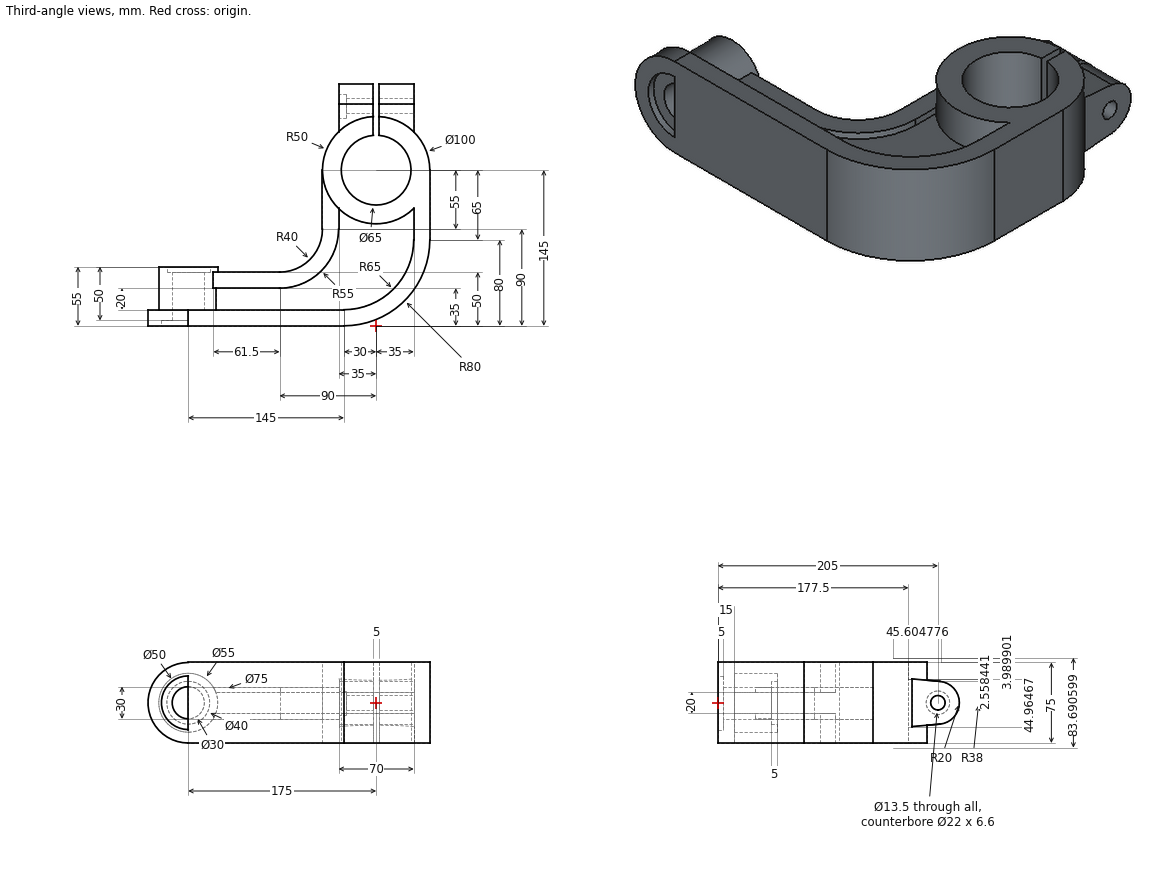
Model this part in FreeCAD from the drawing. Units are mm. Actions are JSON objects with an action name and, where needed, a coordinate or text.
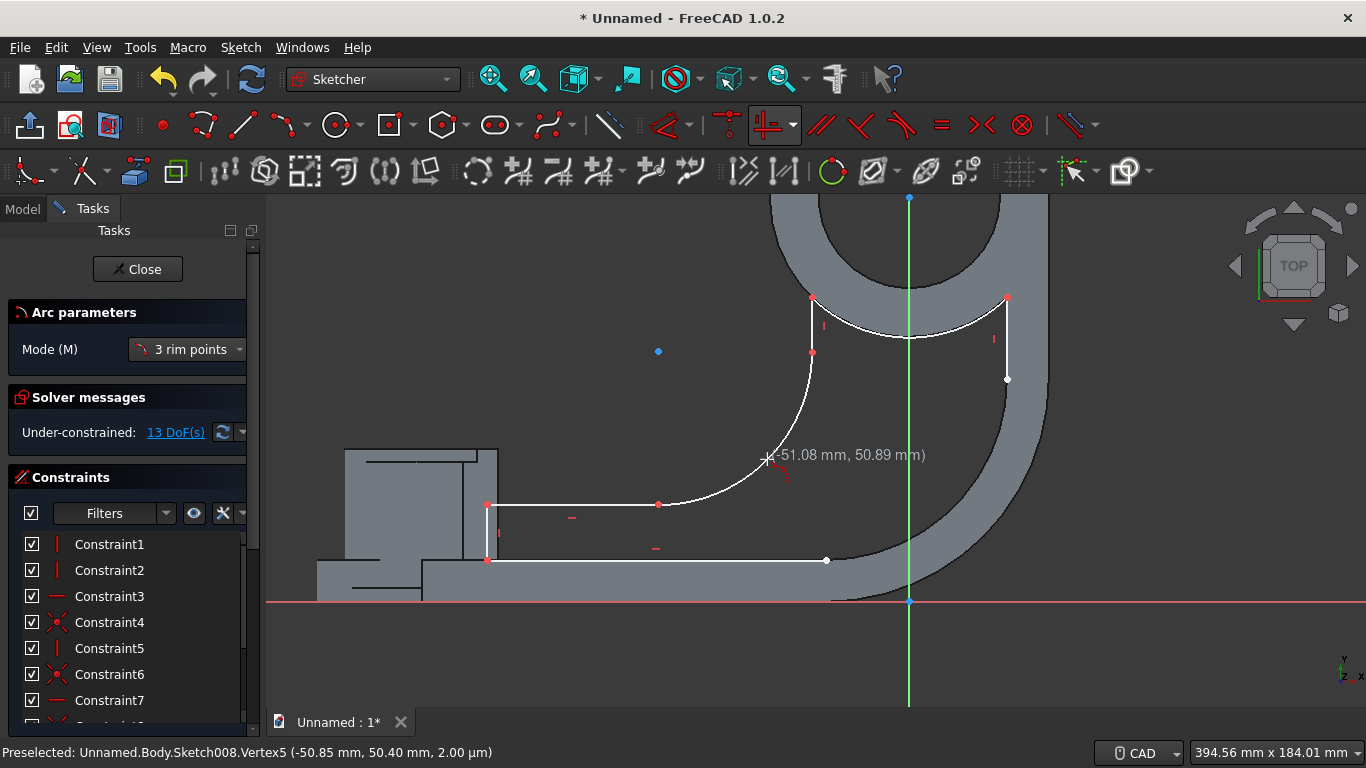
{"action": "left_click", "coordinate": [826, 561]}
{"action": "left_click", "coordinate": [1007, 380]}
{"action": "left_click", "coordinate": [954, 507]}
{"action": "key", "text": "Escape"}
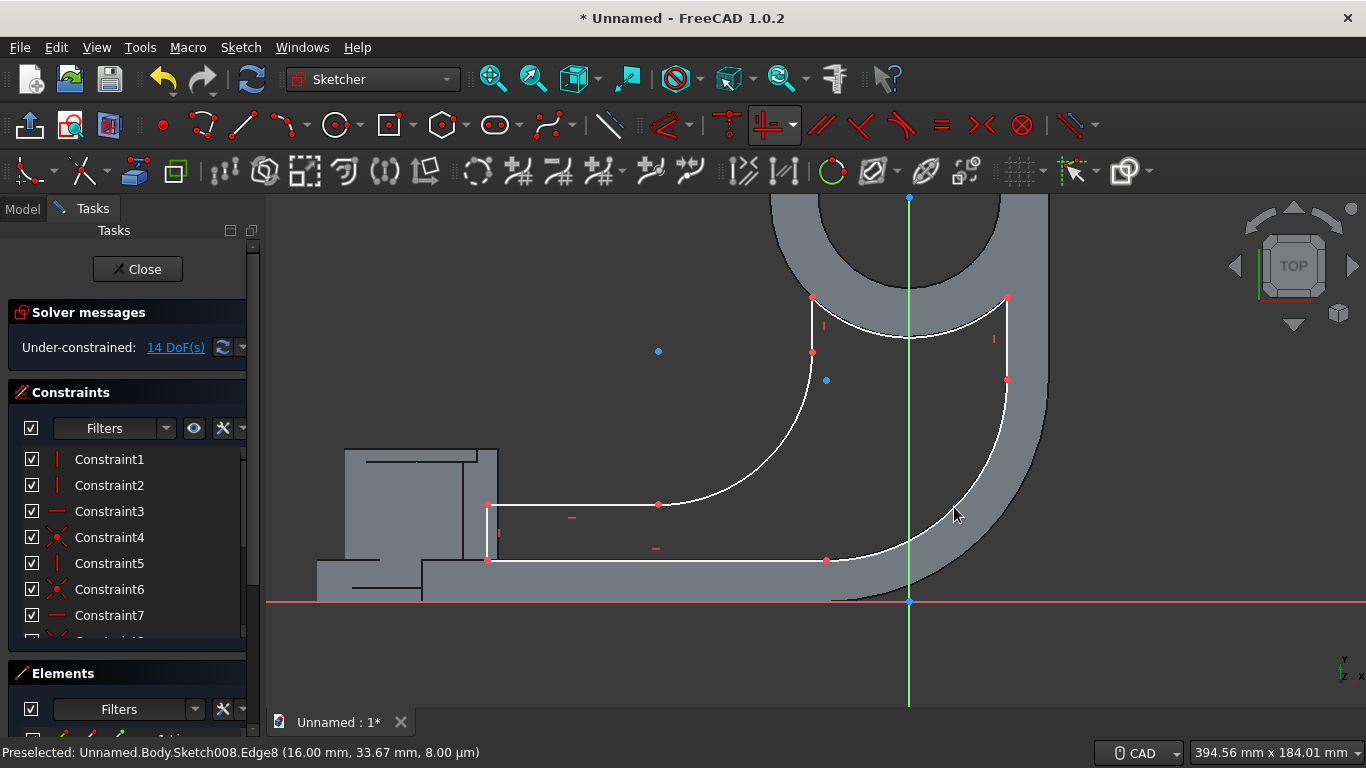
{"action": "scroll", "coordinate": [750, 679], "scroll_direction": "down", "scroll_amount": 1}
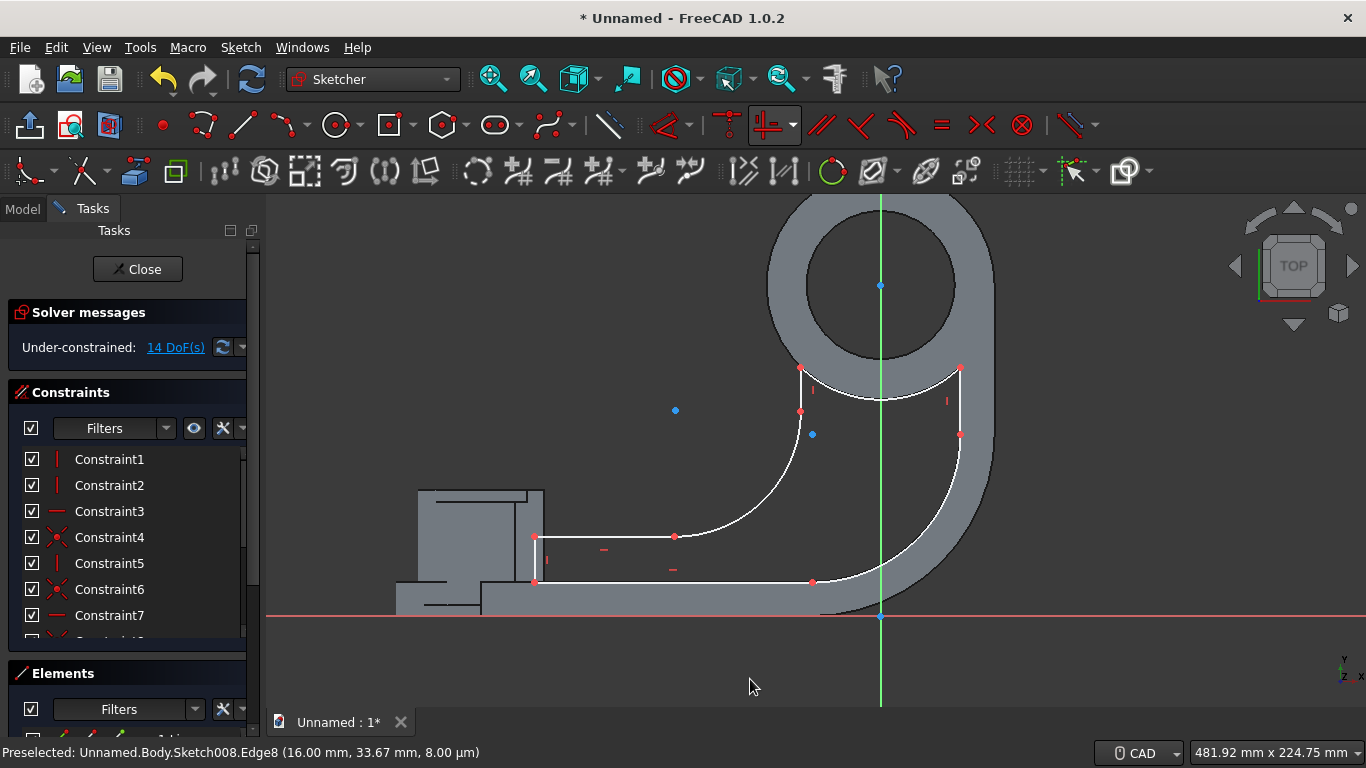
{"action": "left_click", "coordinate": [881, 285]}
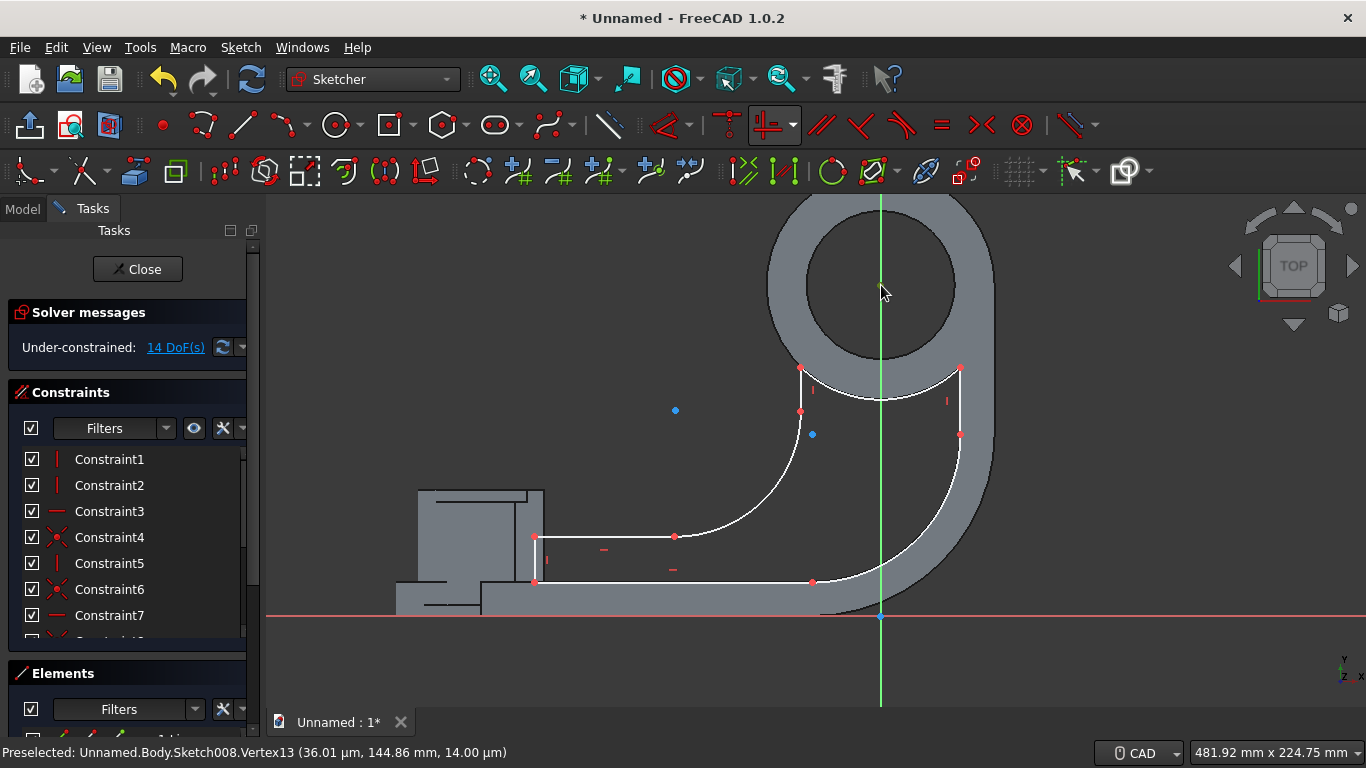
{"action": "left_click", "coordinate": [881, 646]}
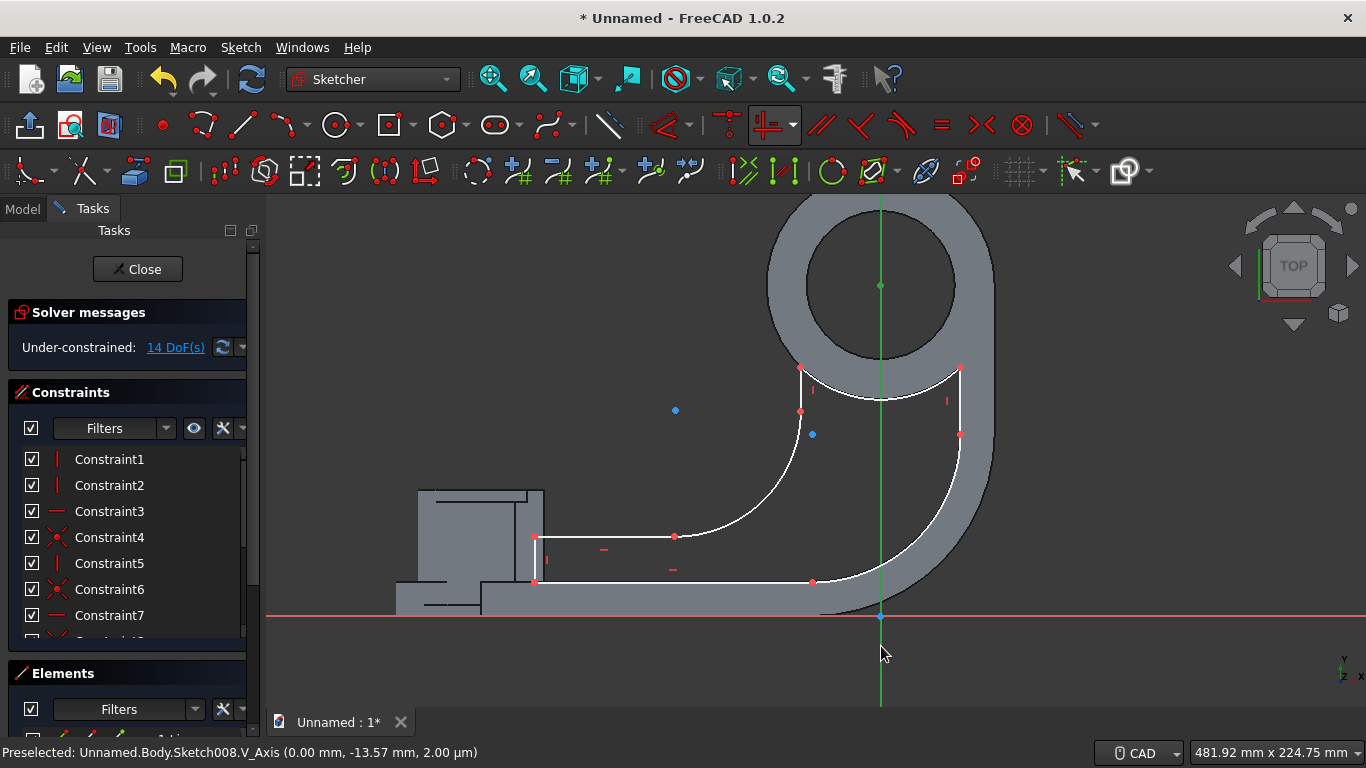
{"action": "key", "text": "c"}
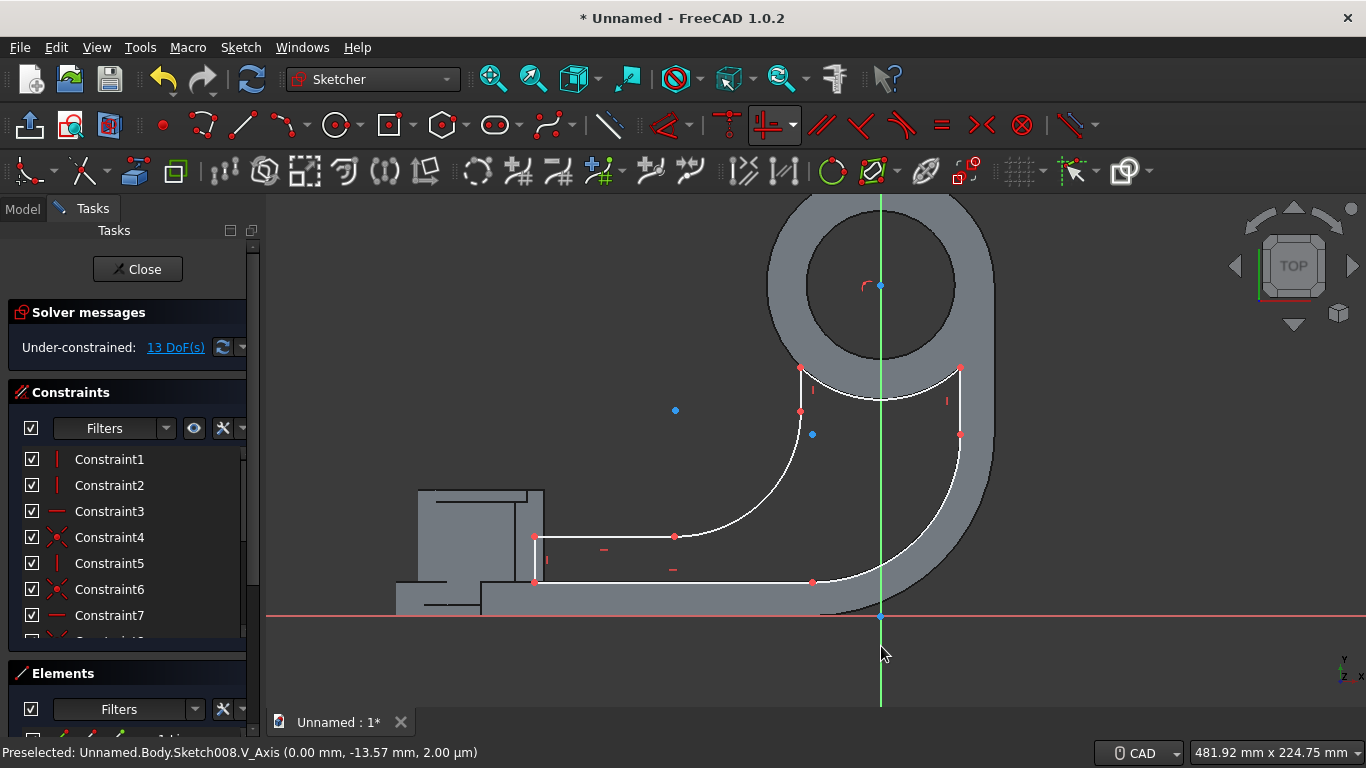
{"action": "left_click", "coordinate": [664, 126]}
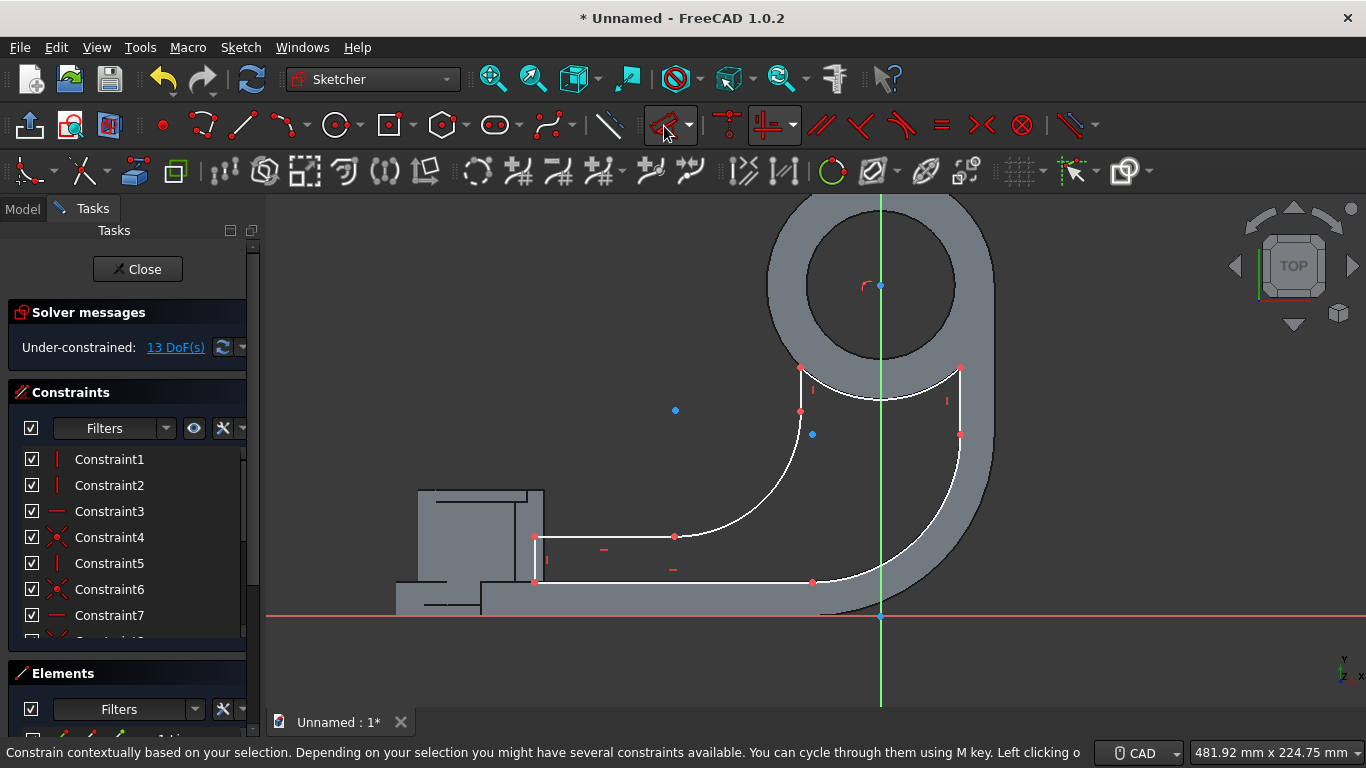
{"action": "left_click", "coordinate": [846, 394]}
{"action": "left_click", "coordinate": [836, 424]}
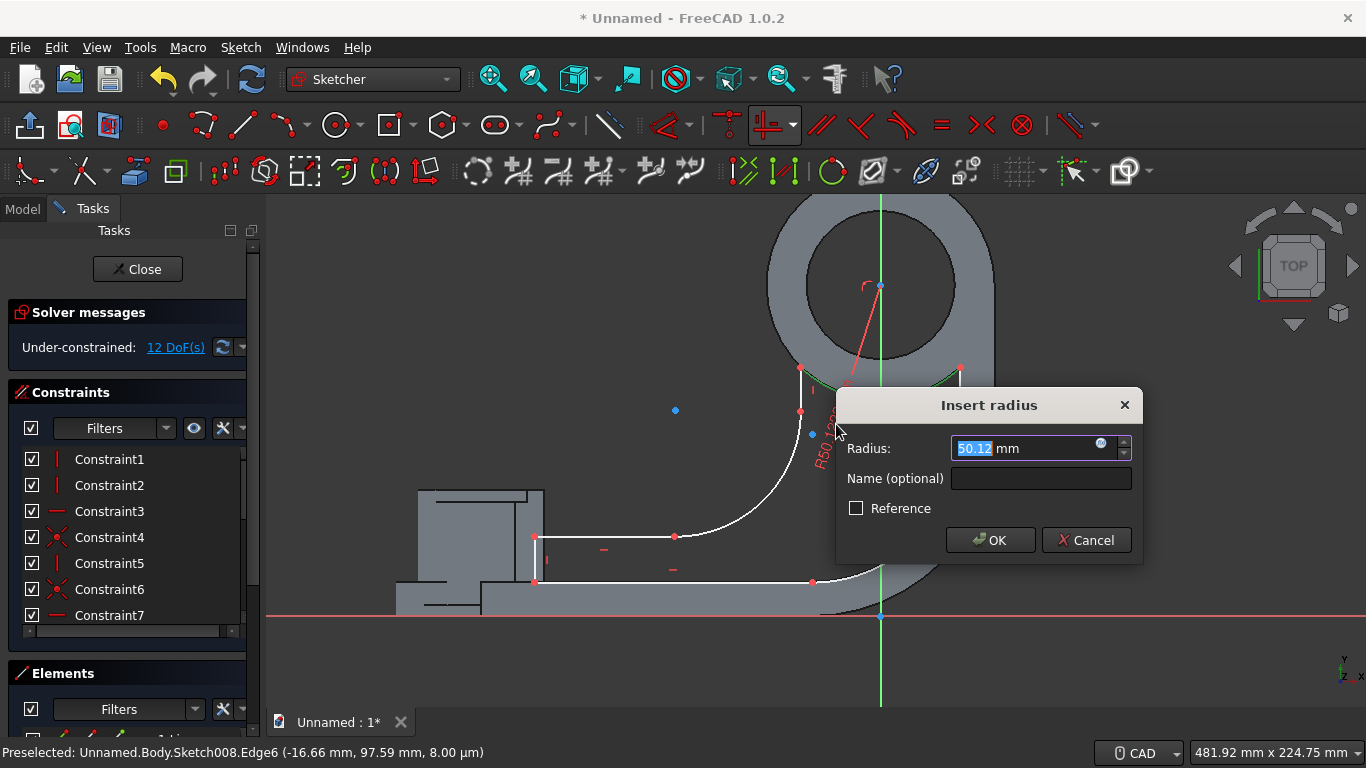
{"action": "type", "text": "50"}
{"action": "key", "text": "Return"}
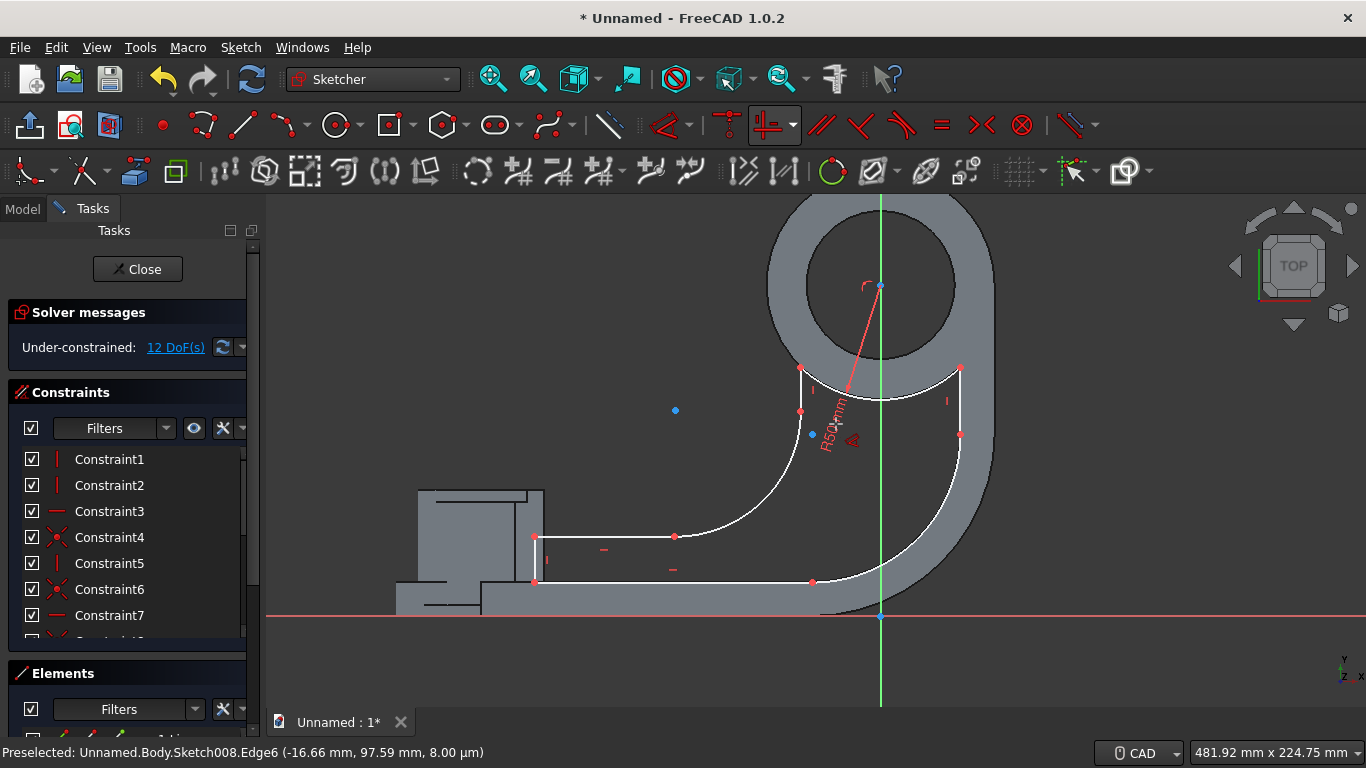
{"action": "left_click", "coordinate": [732, 523]}
{"action": "left_click", "coordinate": [746, 552]}